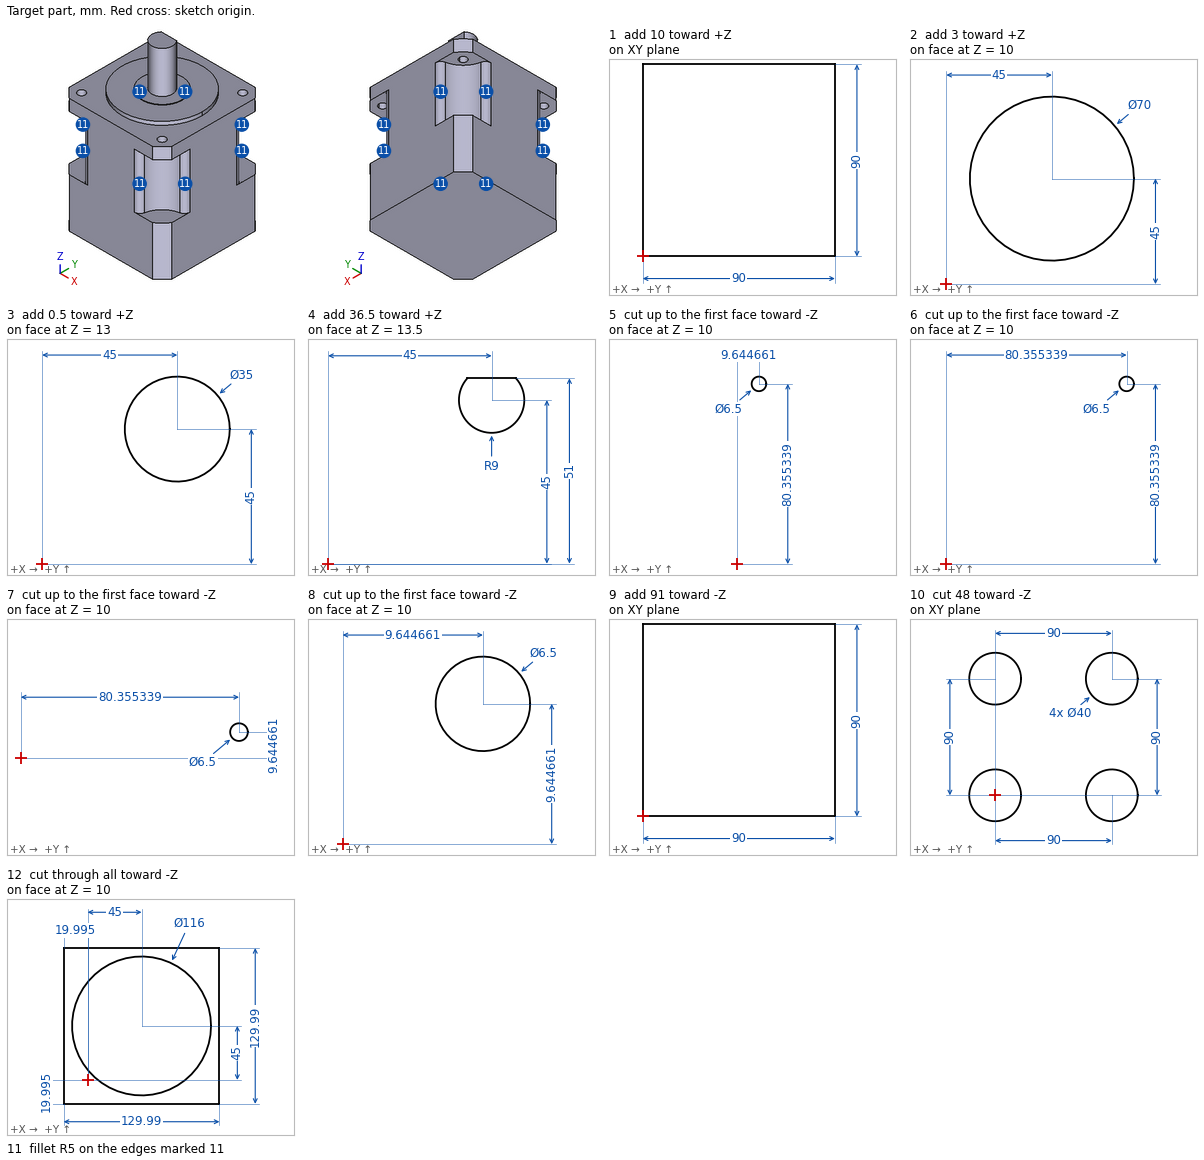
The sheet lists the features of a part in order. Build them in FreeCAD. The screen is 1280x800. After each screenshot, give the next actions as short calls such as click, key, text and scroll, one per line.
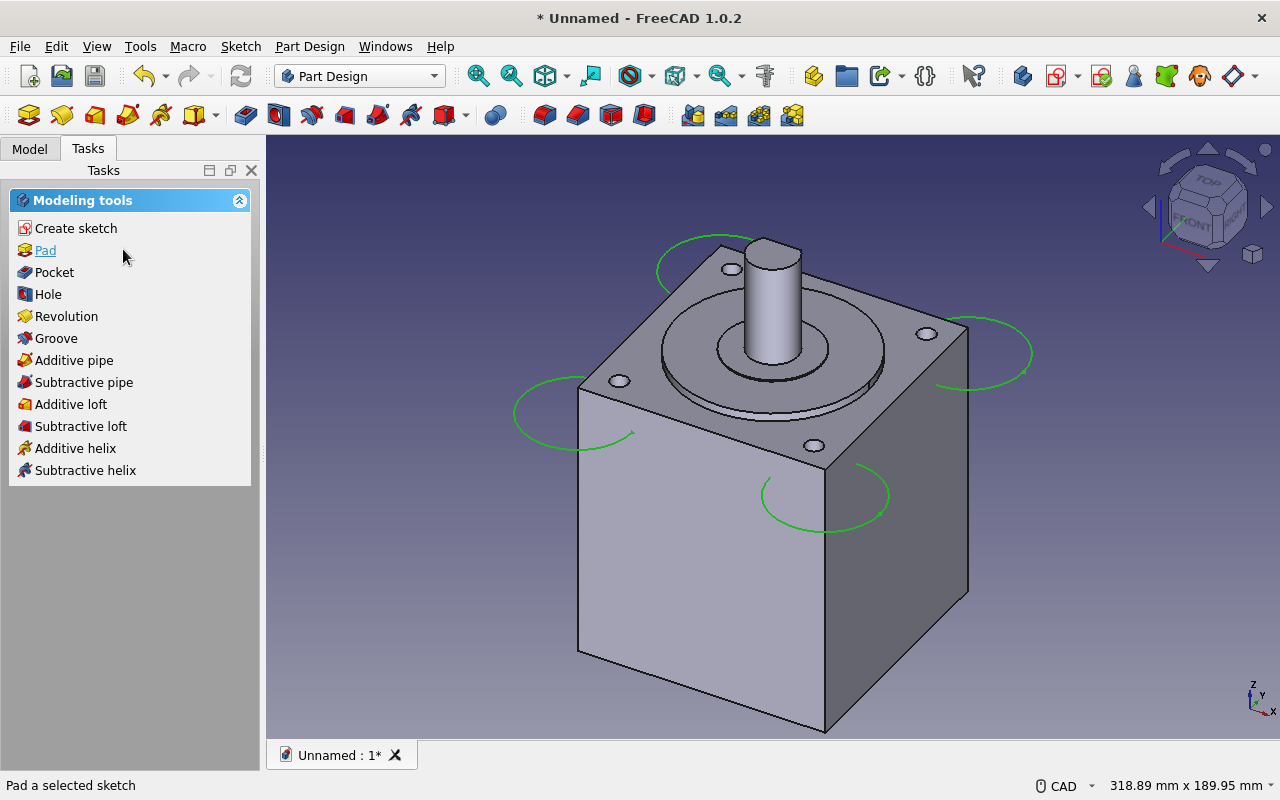
click(246, 116)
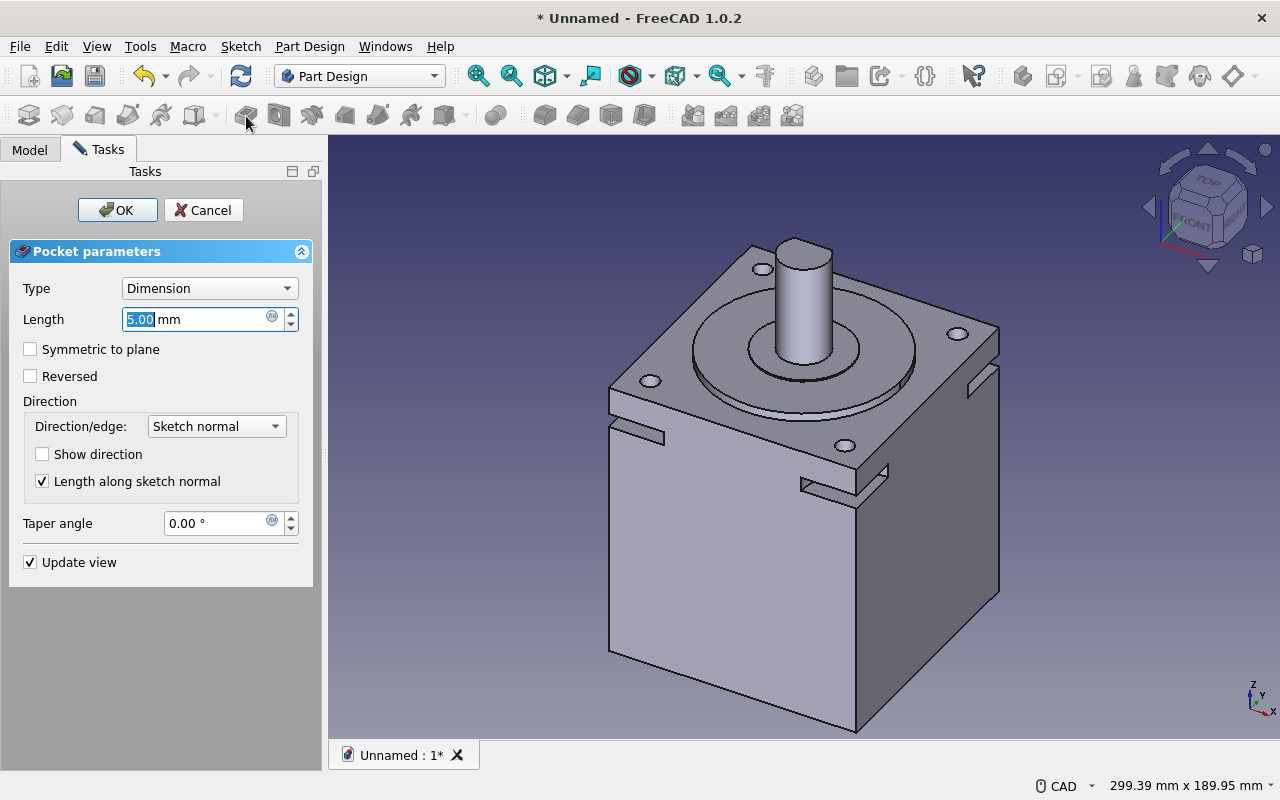
text(48)
key(Tab)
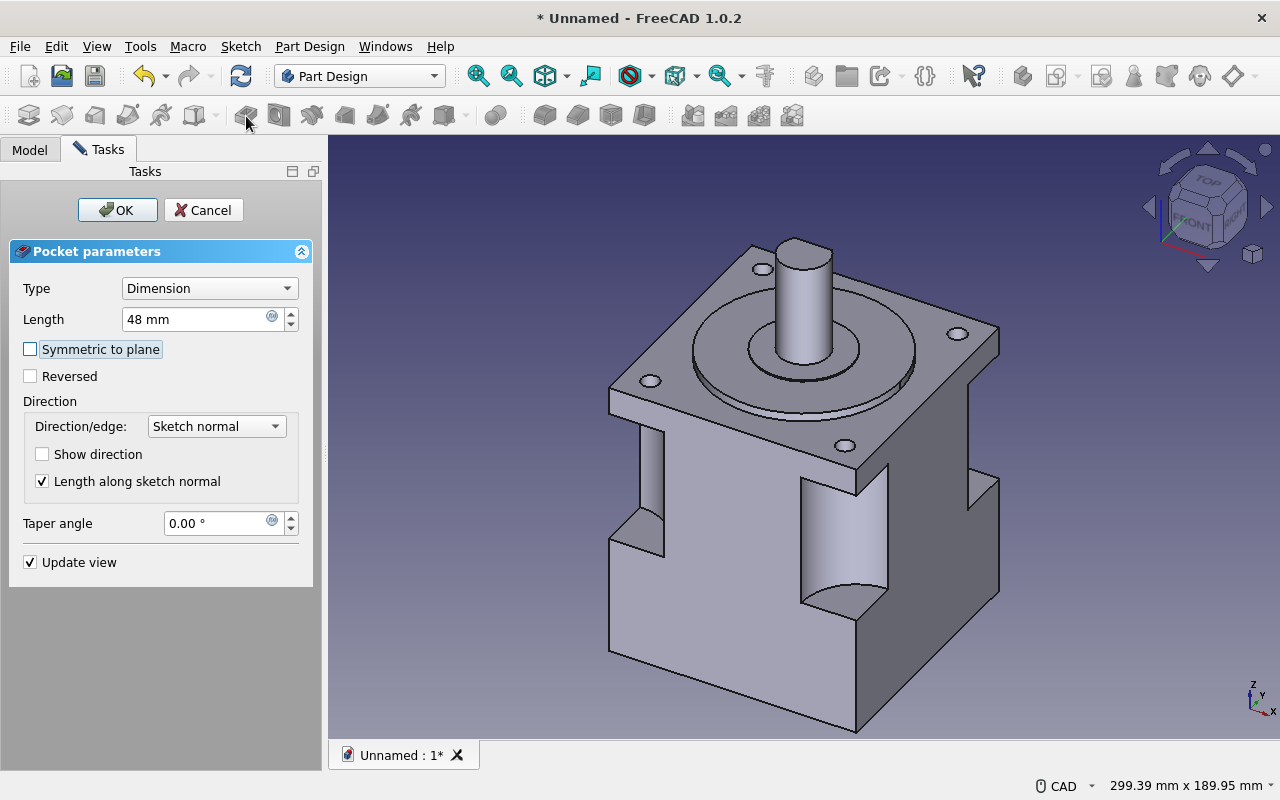
click(118, 210)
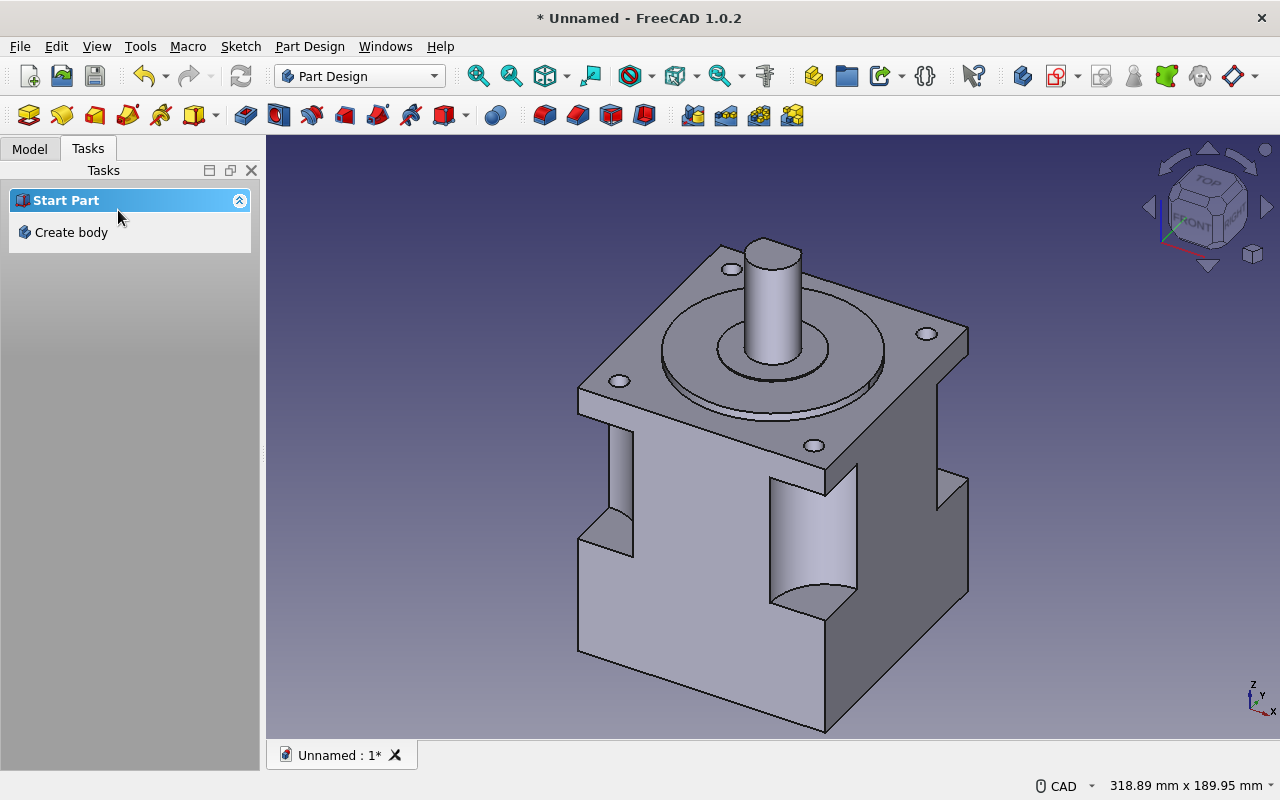
click(770, 539)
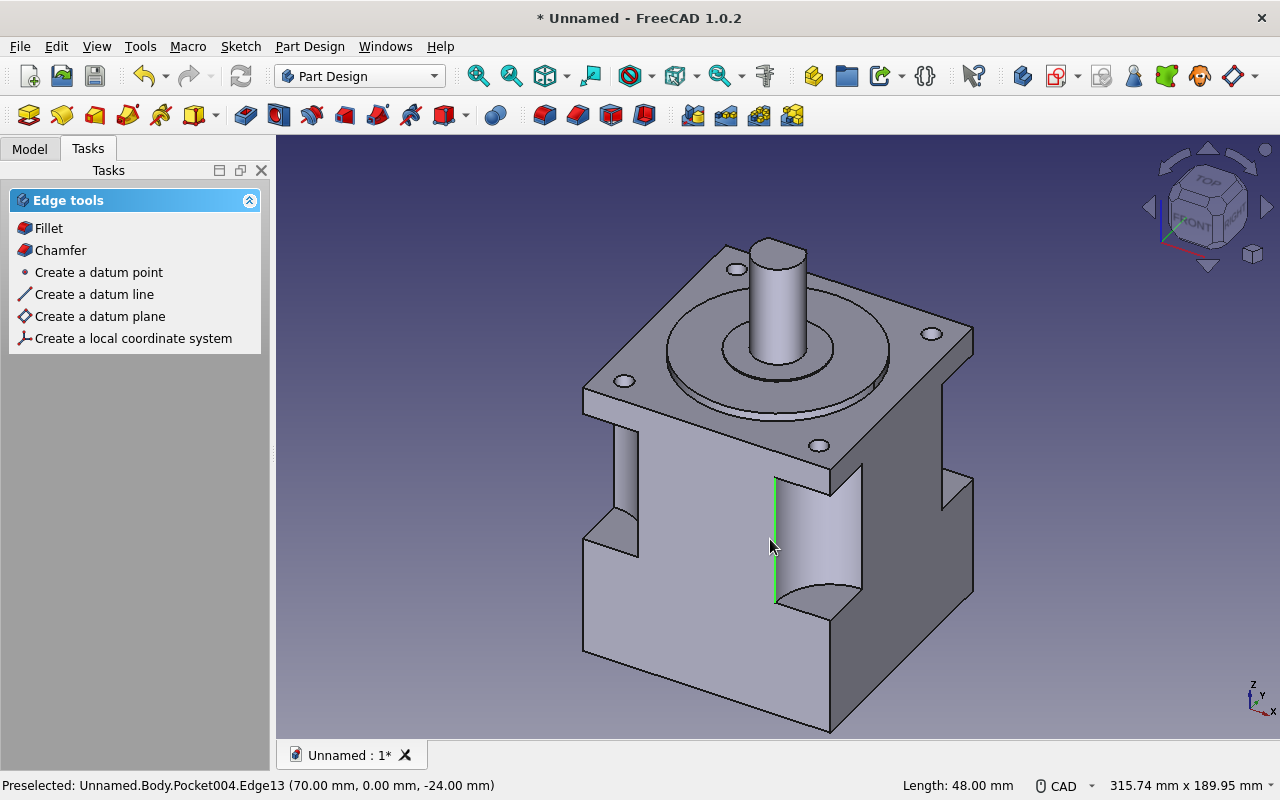
click(862, 526, ctrl)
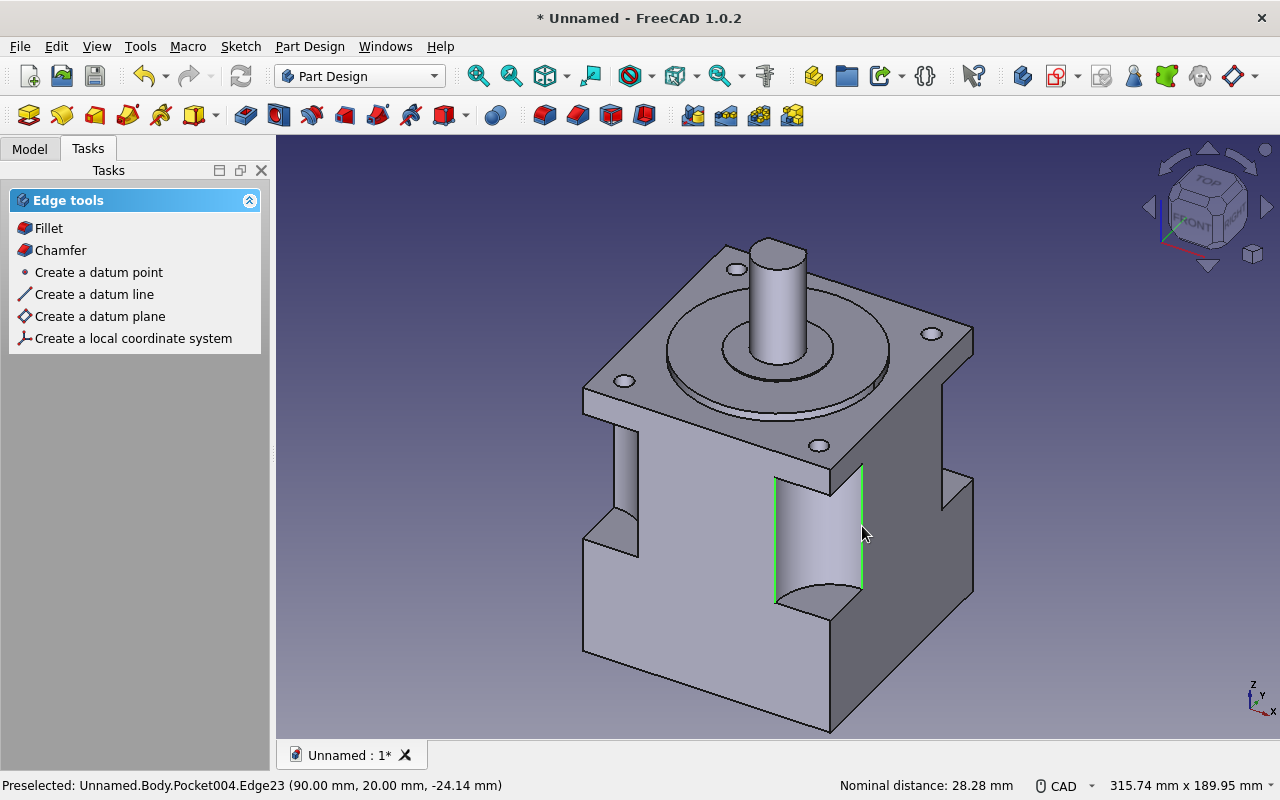
key(0)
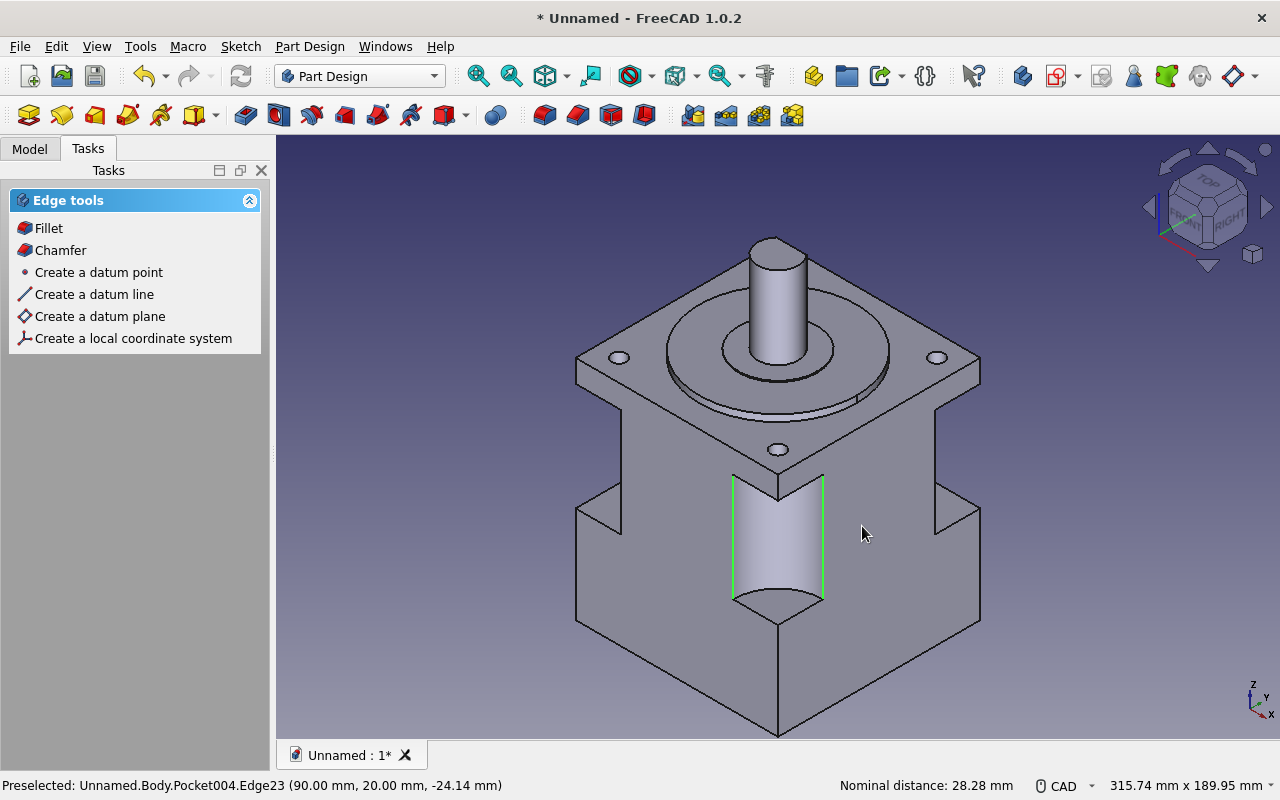
key(2)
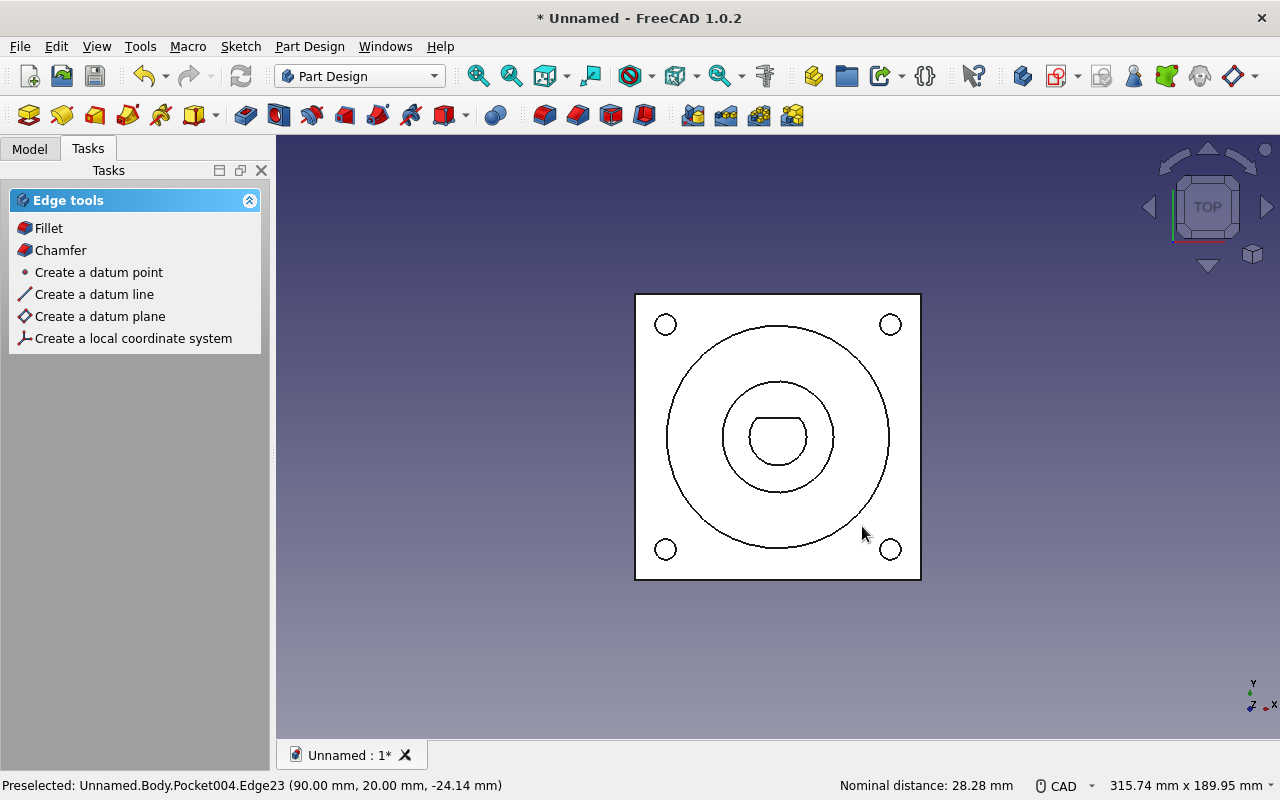
key(1)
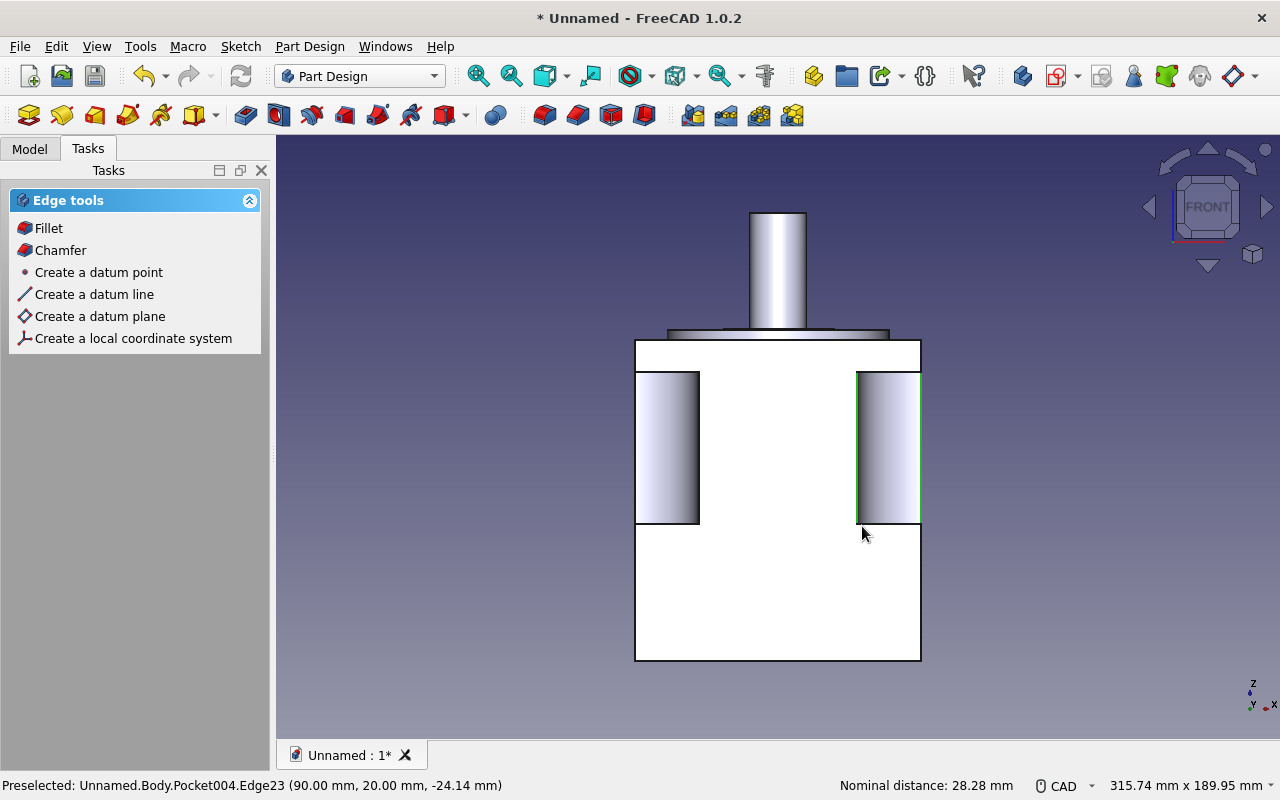
click(699, 447, ctrl)